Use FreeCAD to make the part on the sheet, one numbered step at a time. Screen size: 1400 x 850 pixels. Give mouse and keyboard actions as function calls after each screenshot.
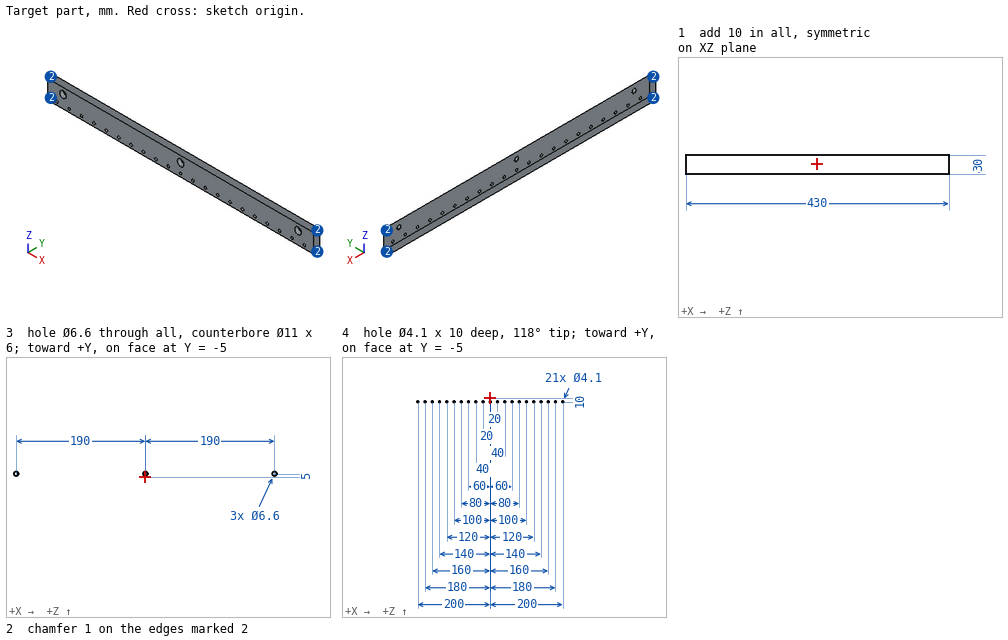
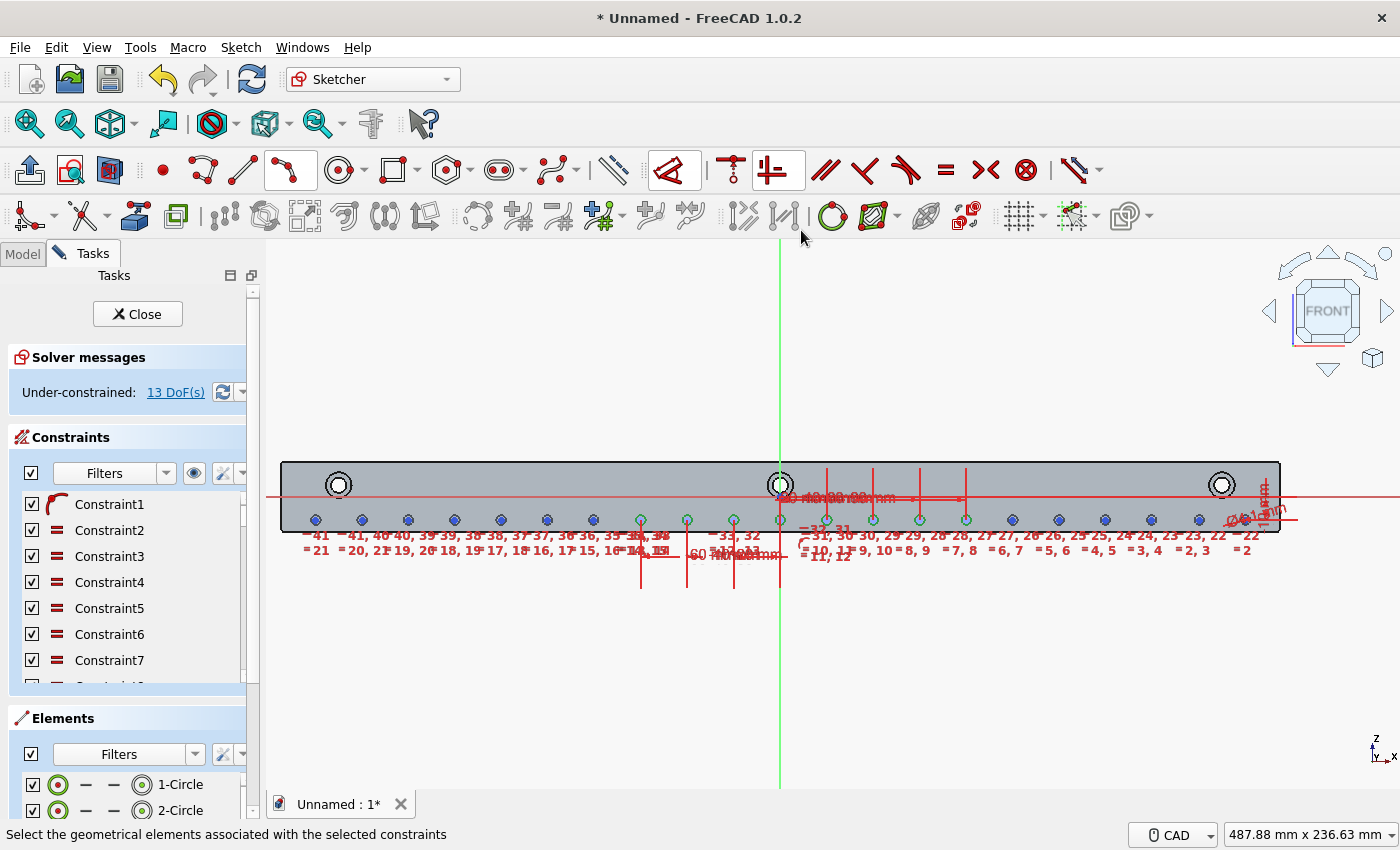
click(594, 520)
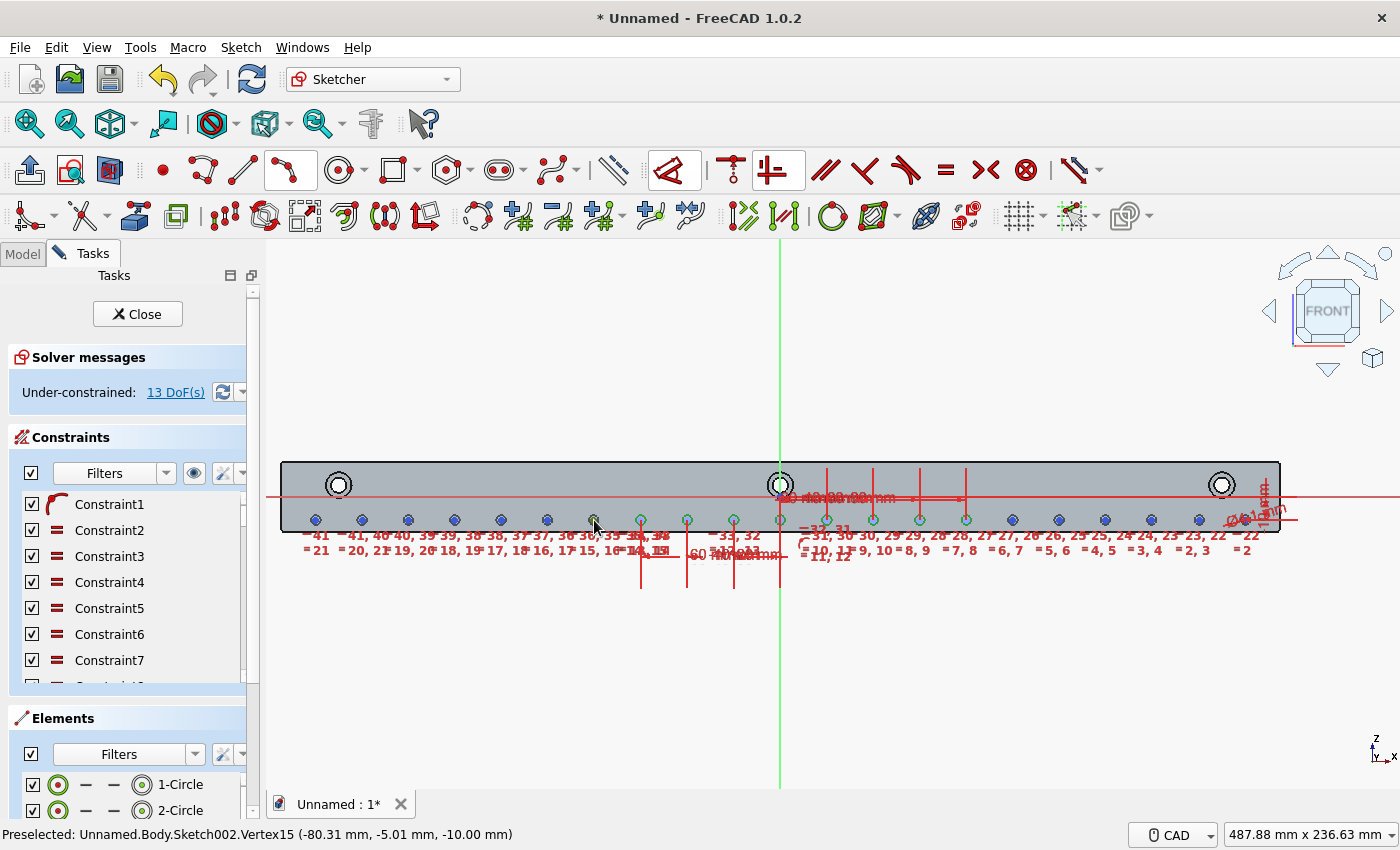
click(696, 170)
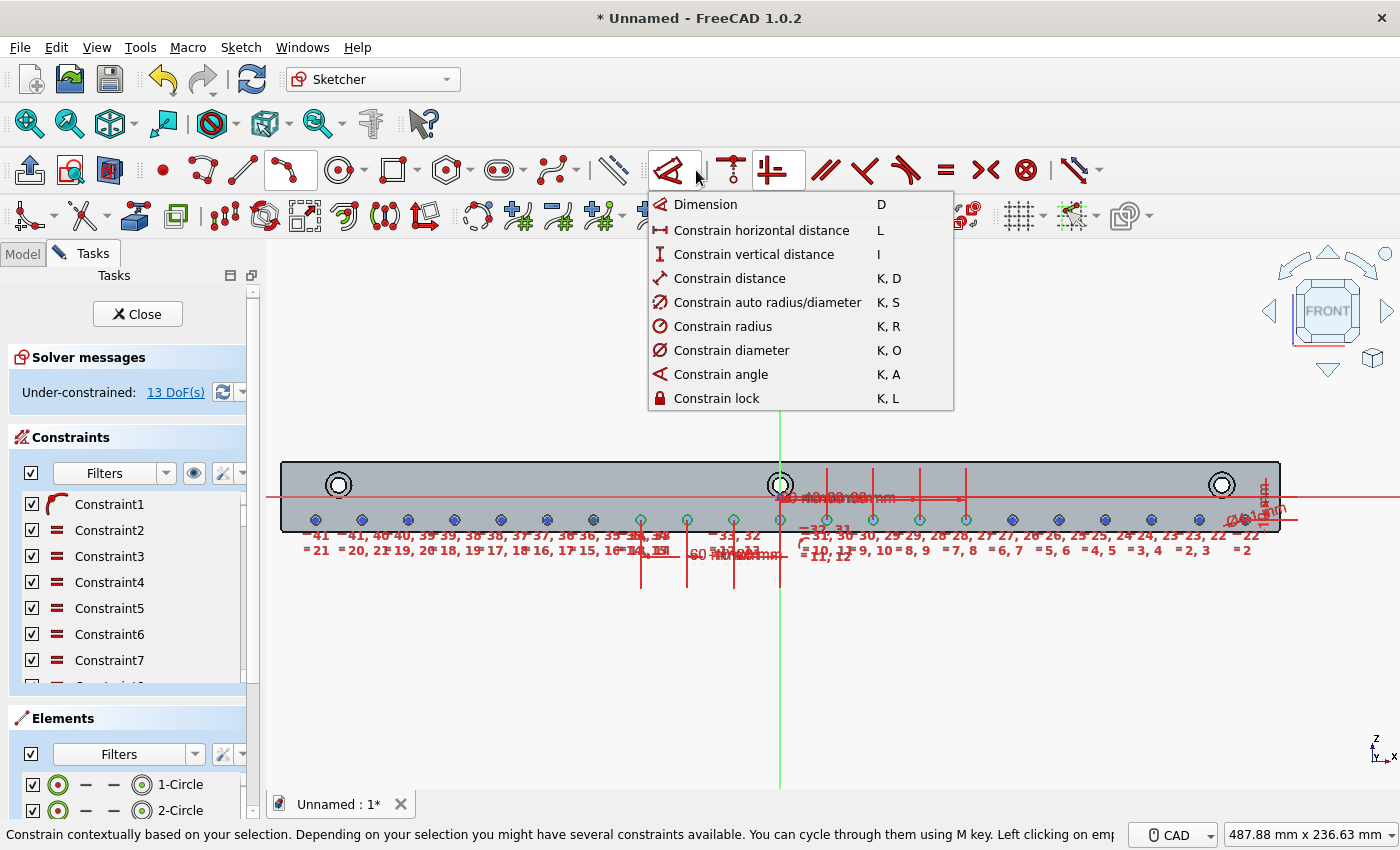
click(801, 230)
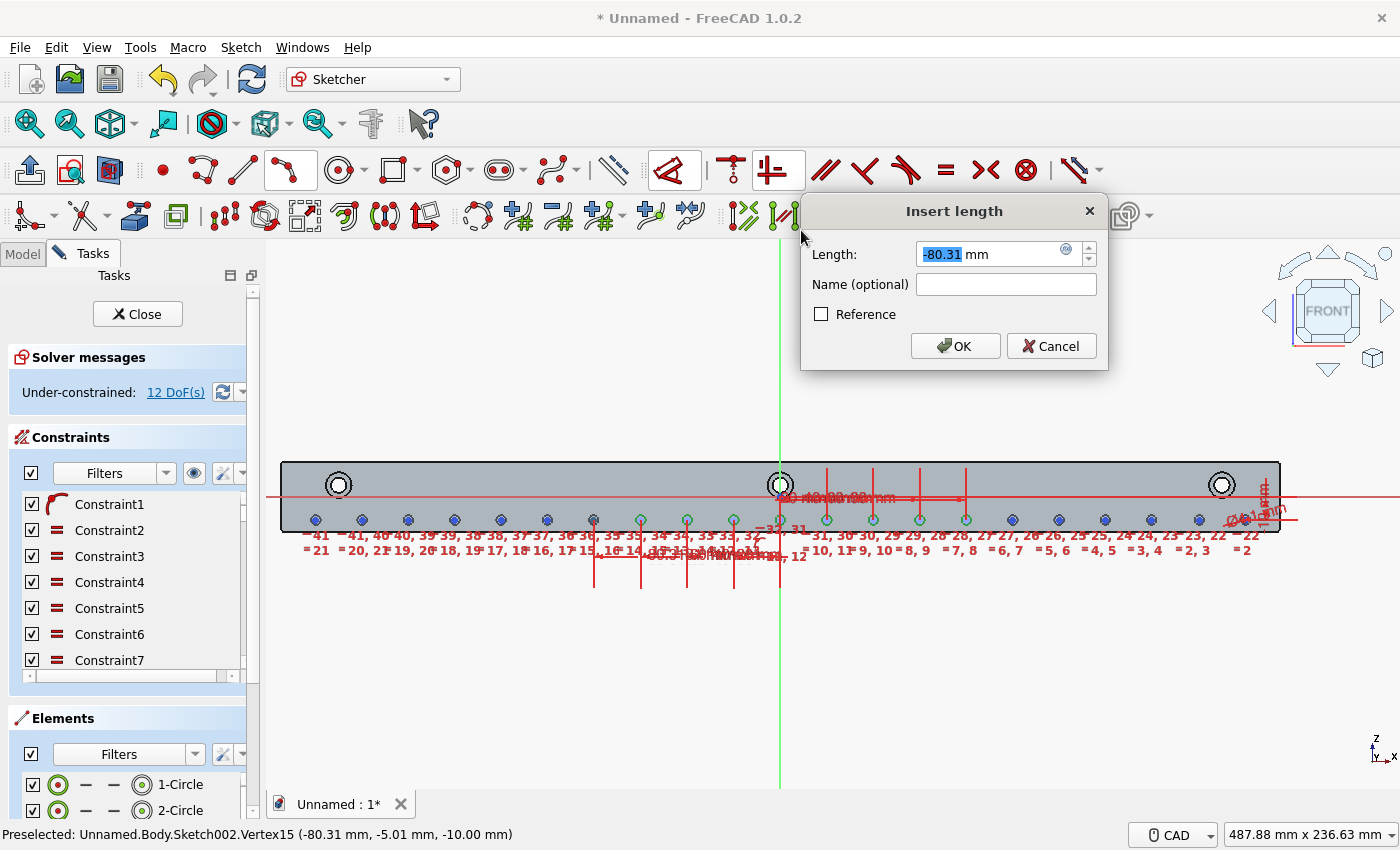
text(-80)
key(Return)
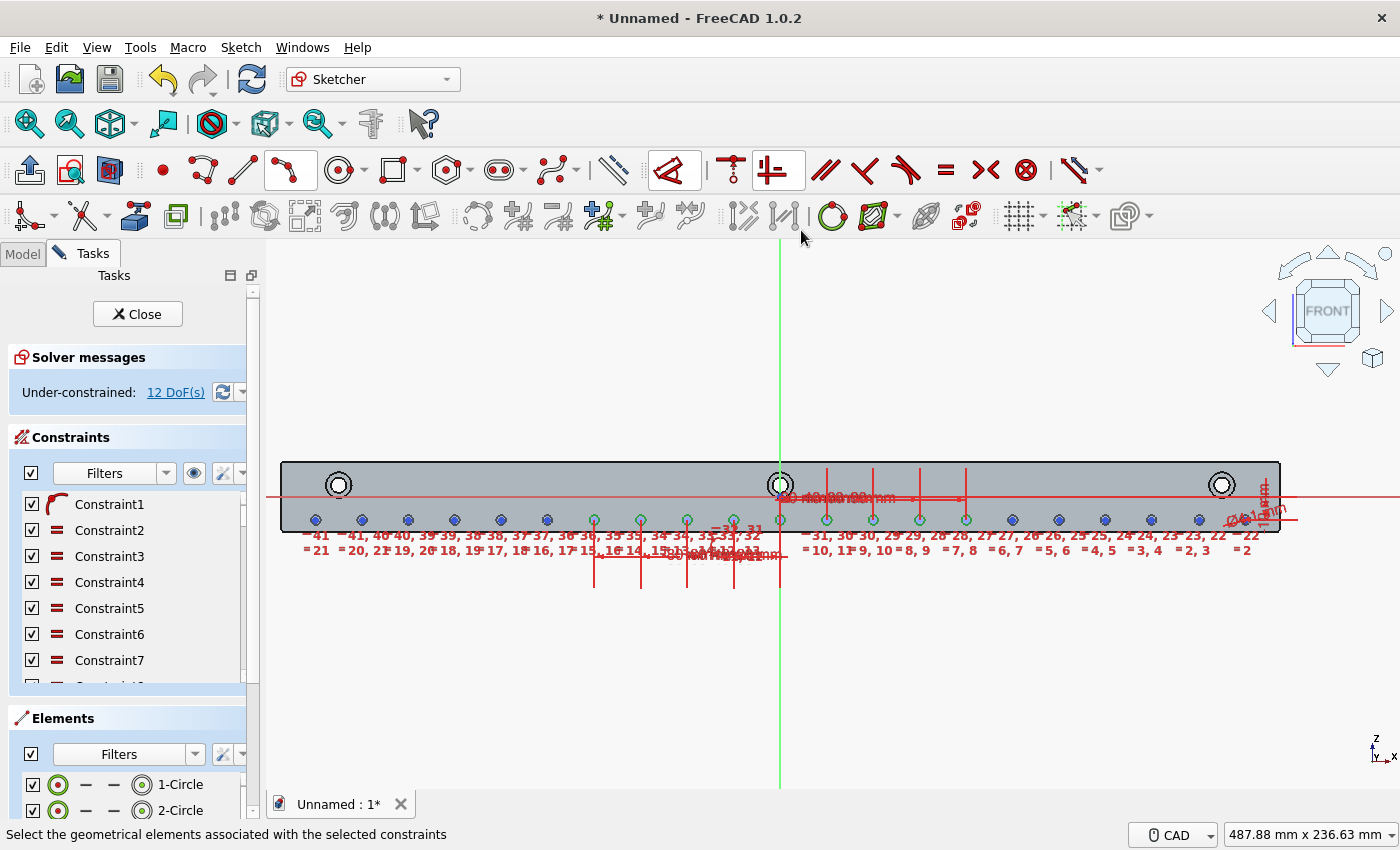
scroll(732, 521, down, 2)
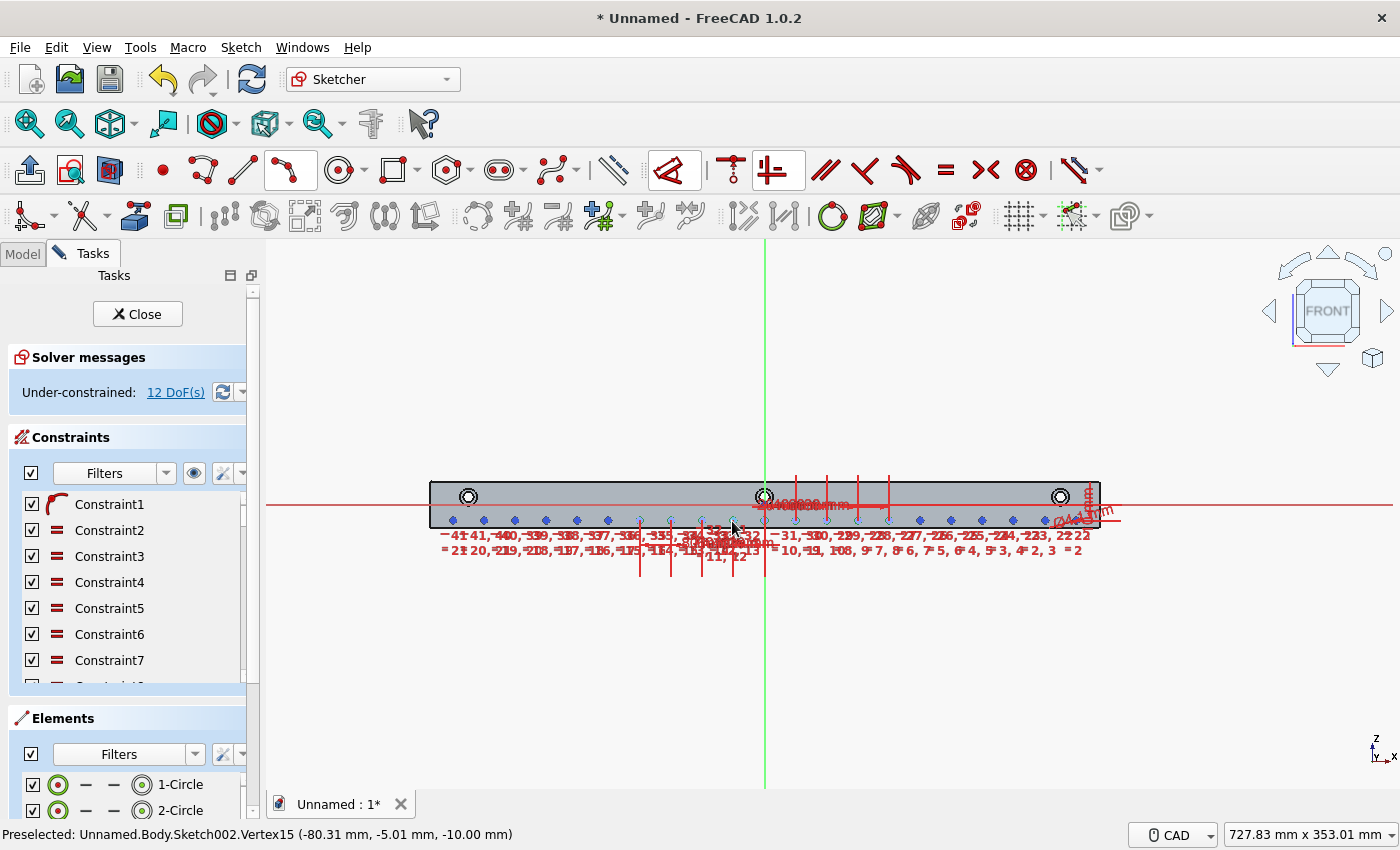
click(1076, 521)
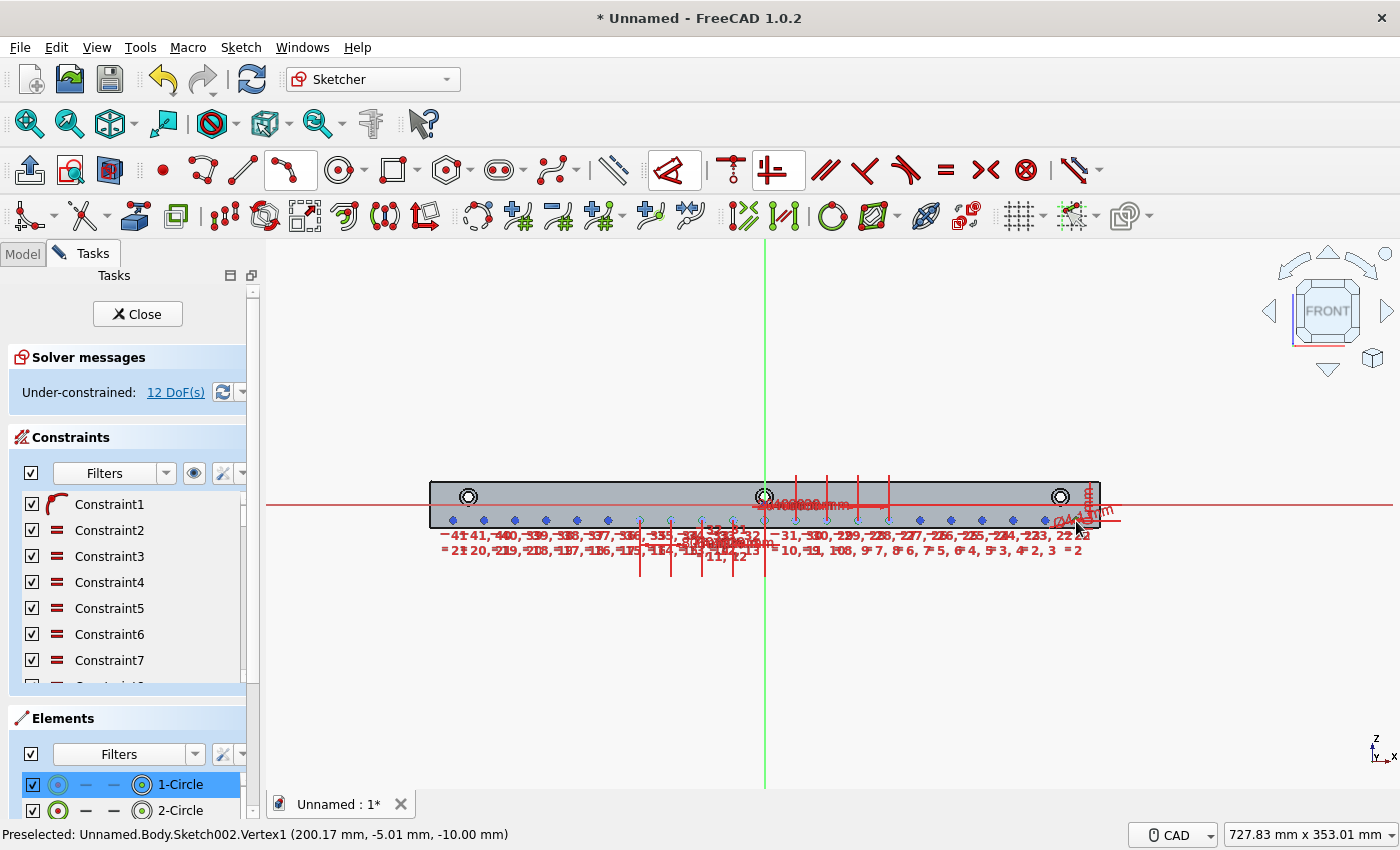
click(696, 170)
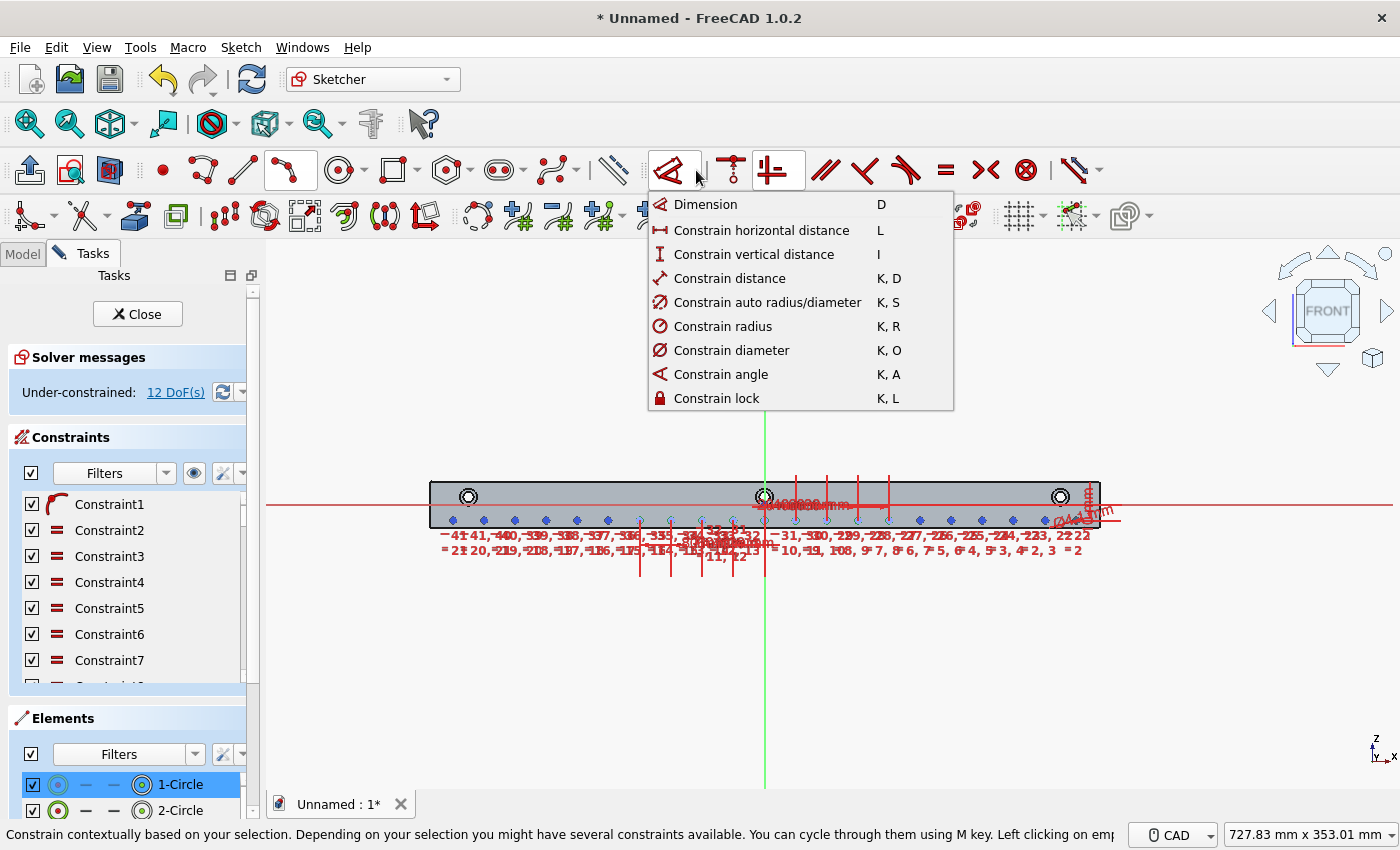
click(801, 230)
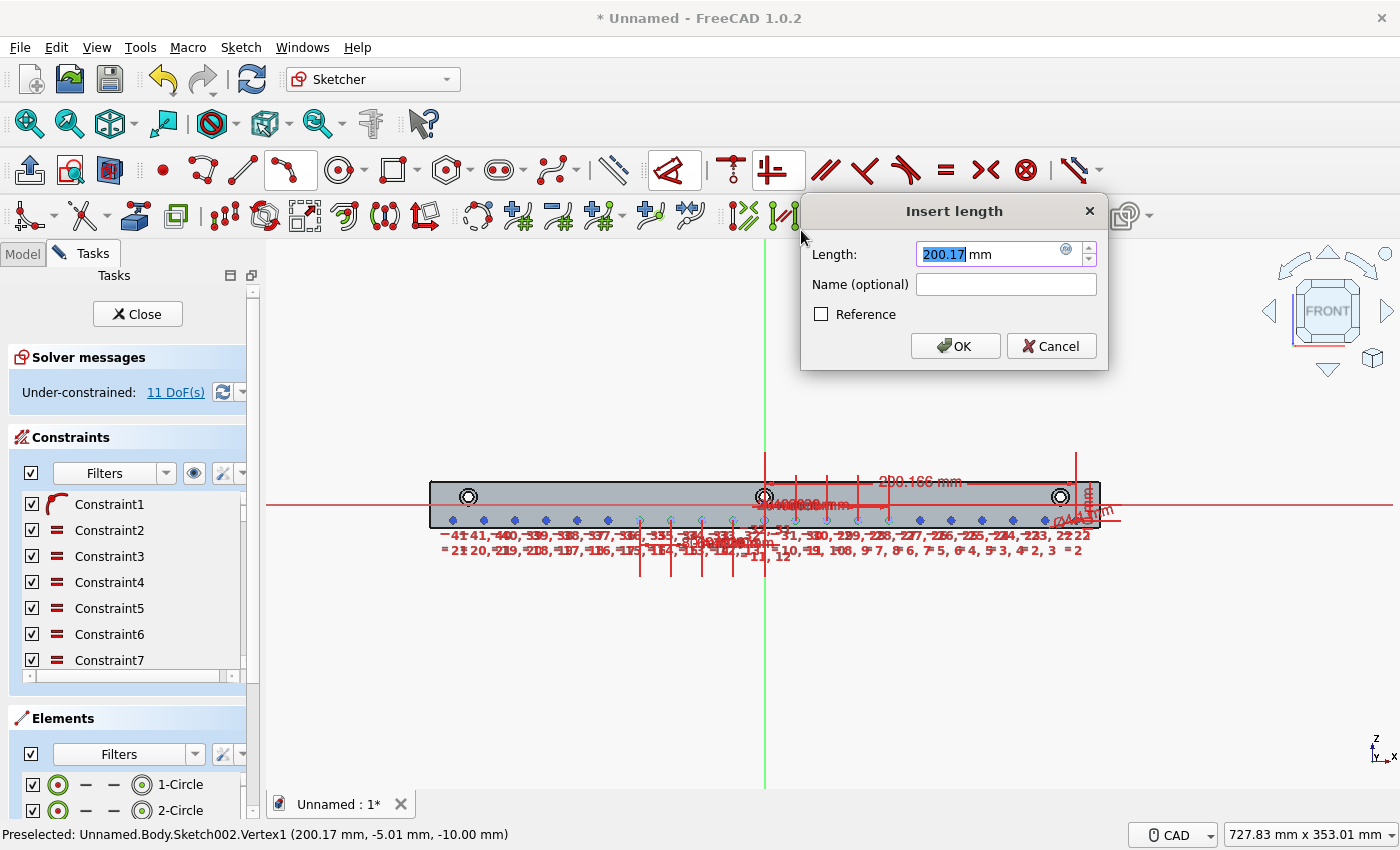
text(200)
key(Return)